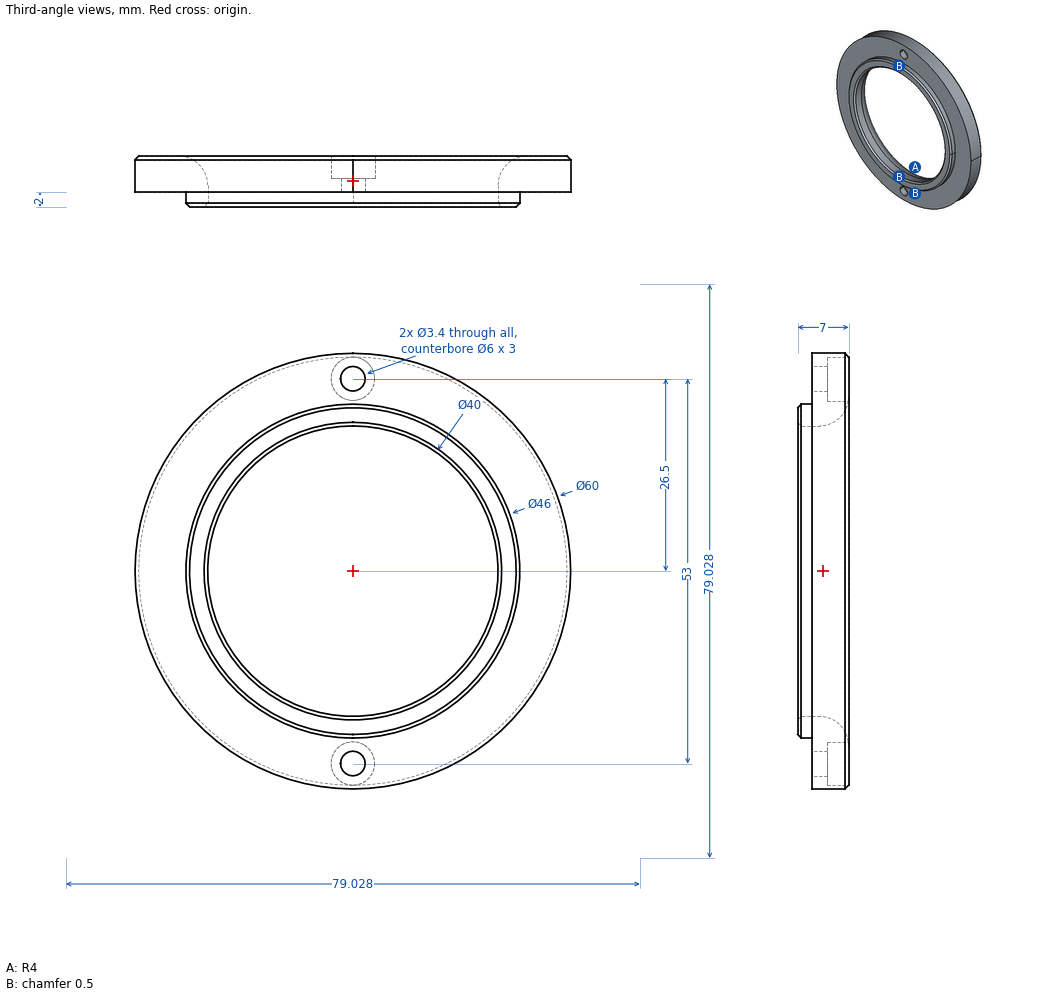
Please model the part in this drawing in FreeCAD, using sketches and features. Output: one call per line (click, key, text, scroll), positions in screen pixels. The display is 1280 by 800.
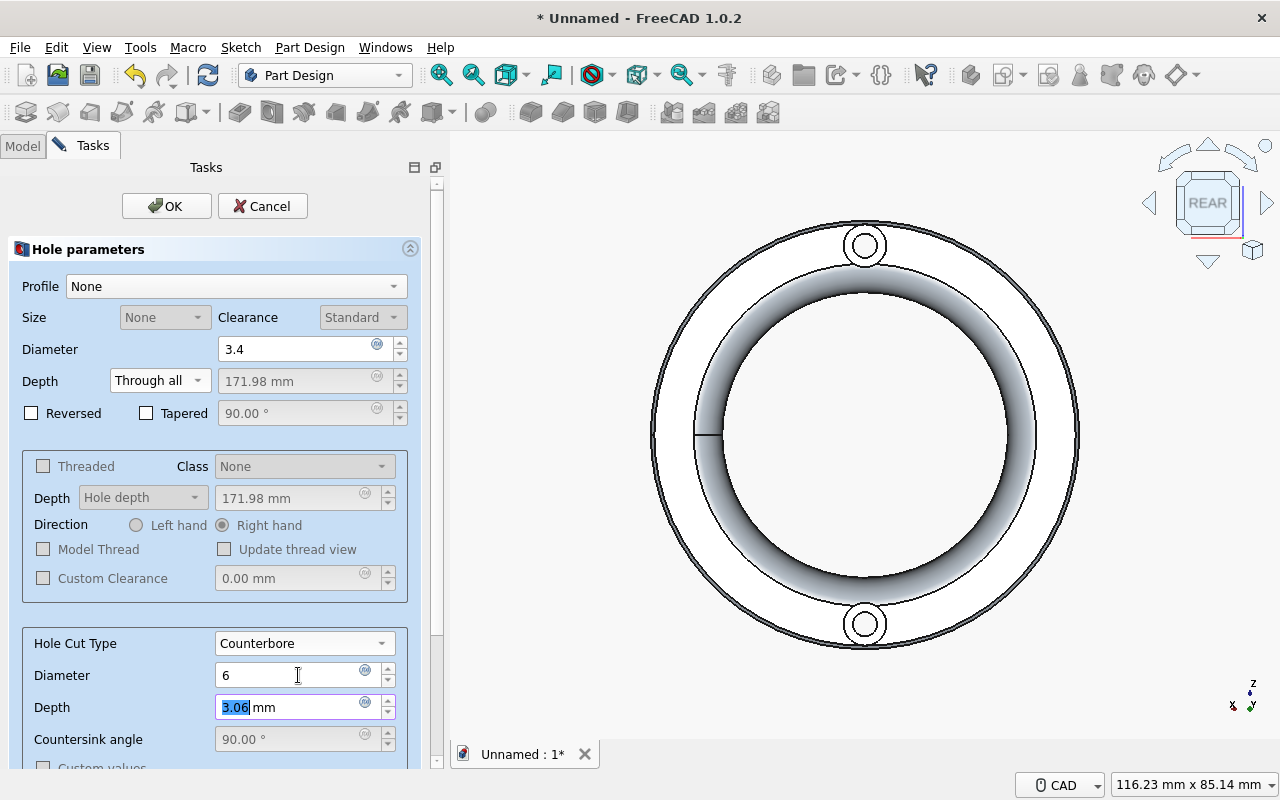
text(3)
key(Tab)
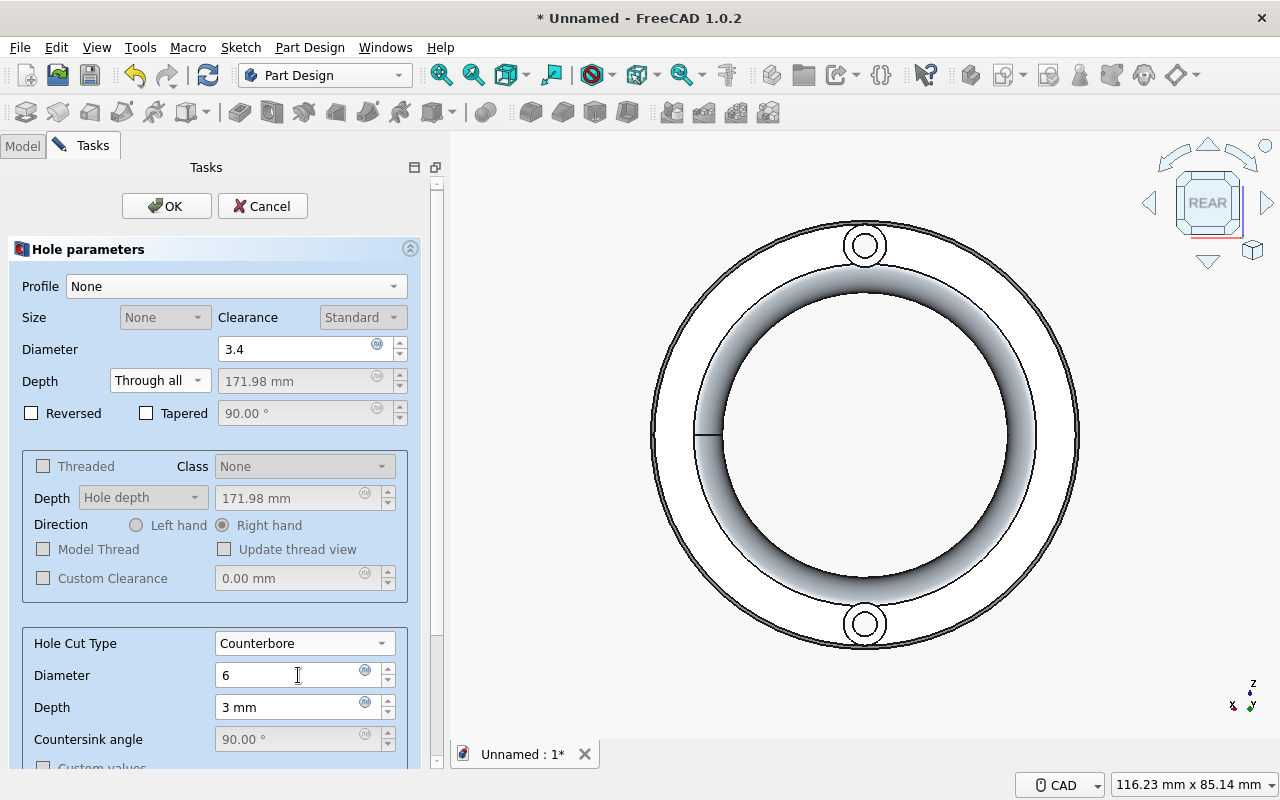
click(167, 206)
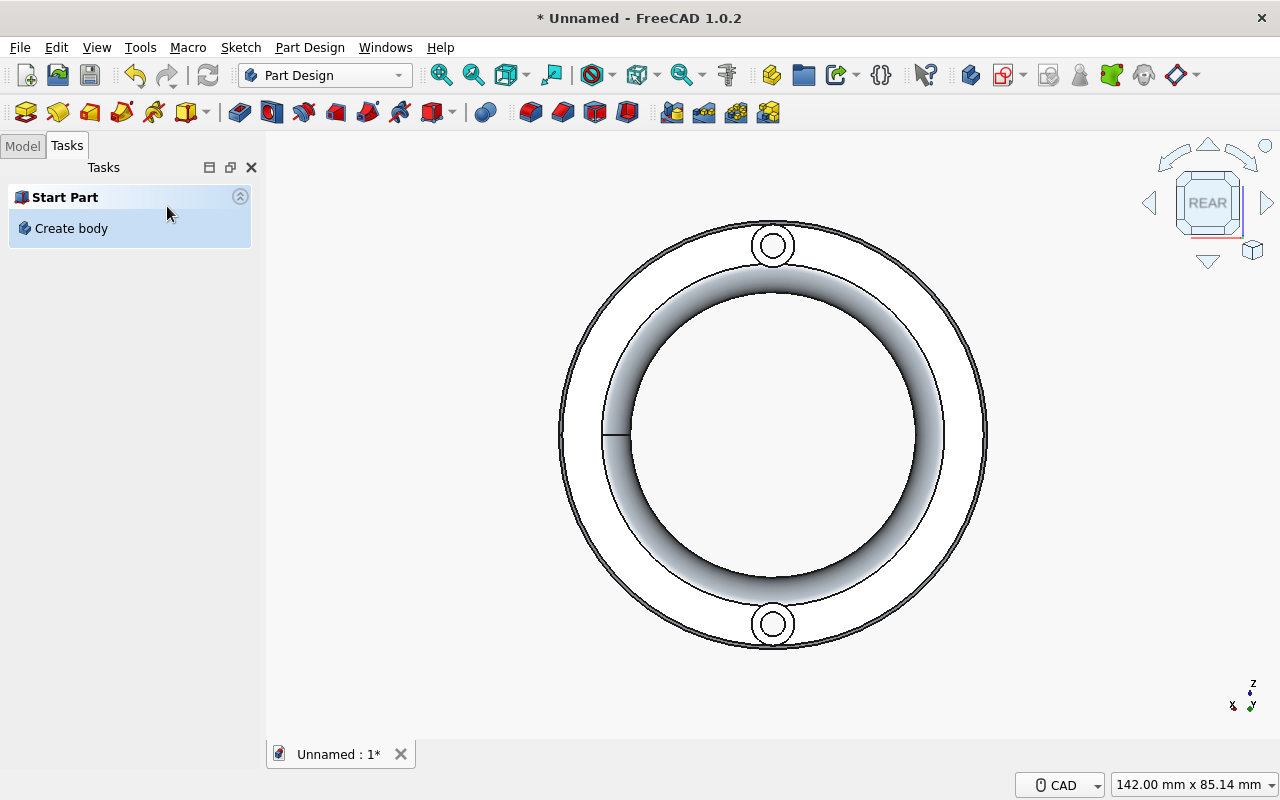
key(0)